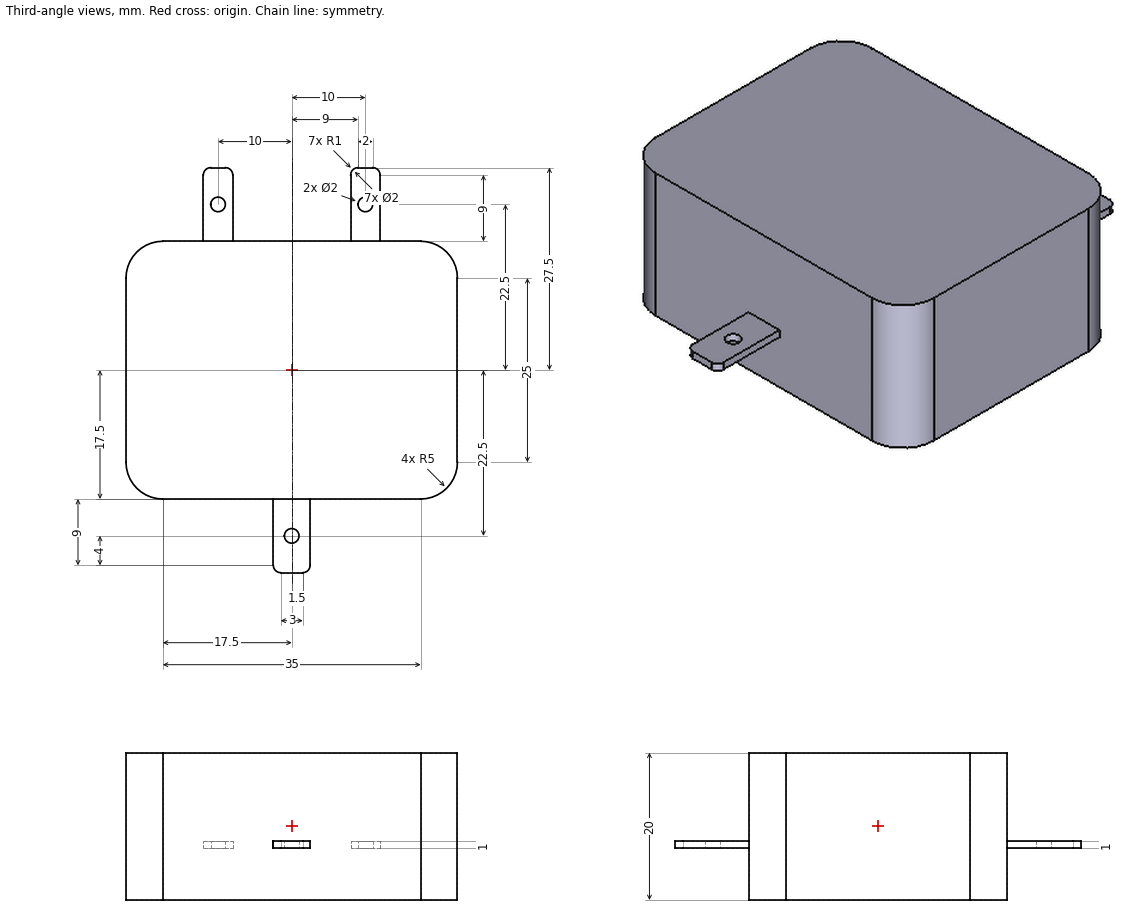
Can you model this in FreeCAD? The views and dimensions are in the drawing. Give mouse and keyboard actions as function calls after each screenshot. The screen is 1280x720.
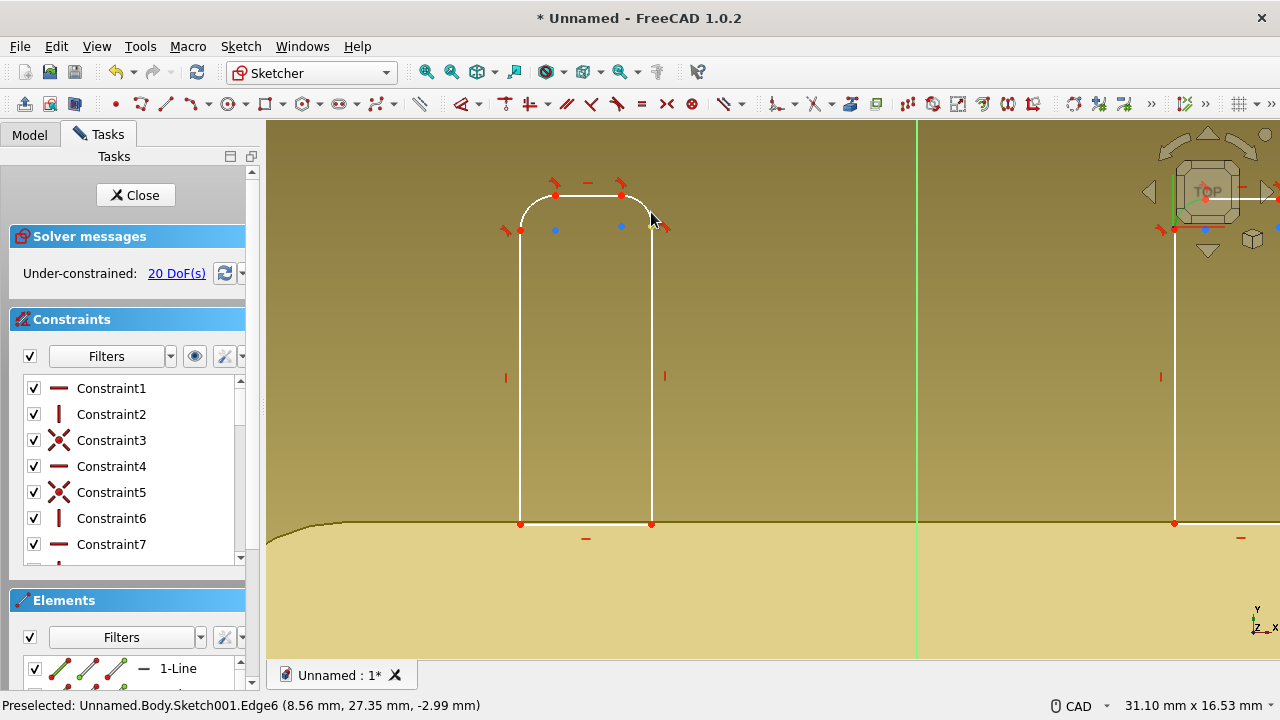
click(649, 212)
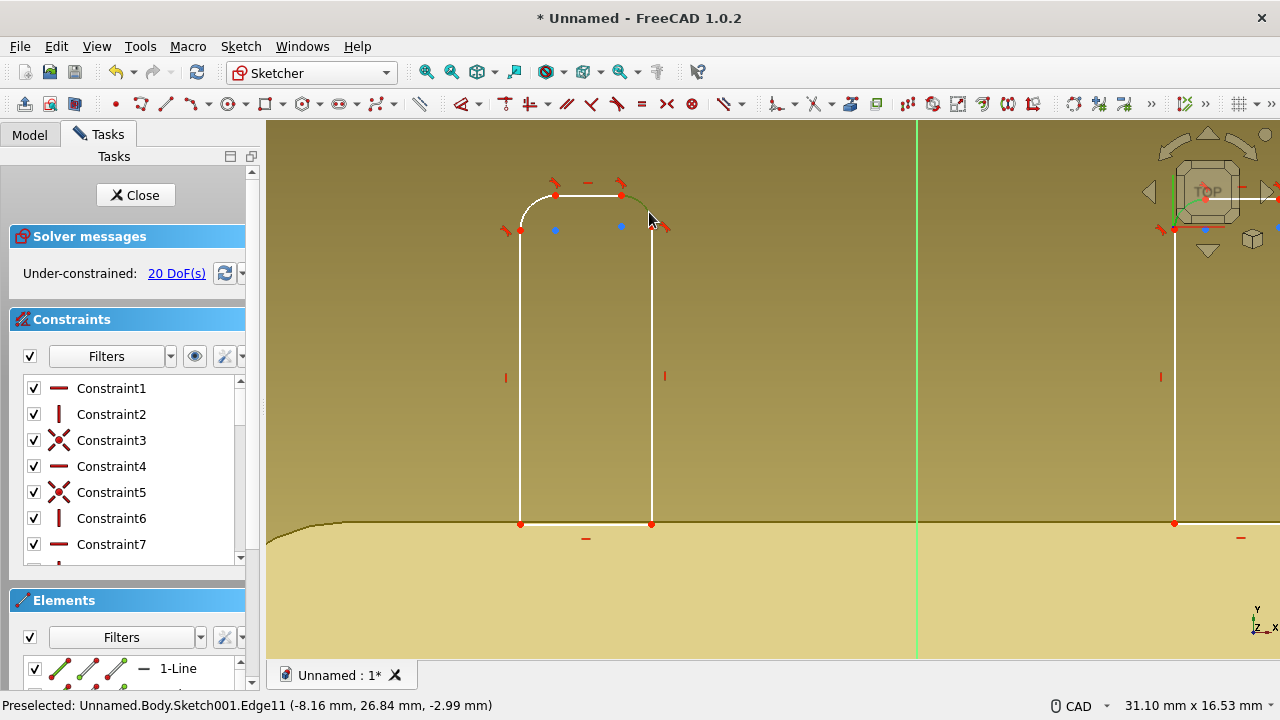
click(540, 200)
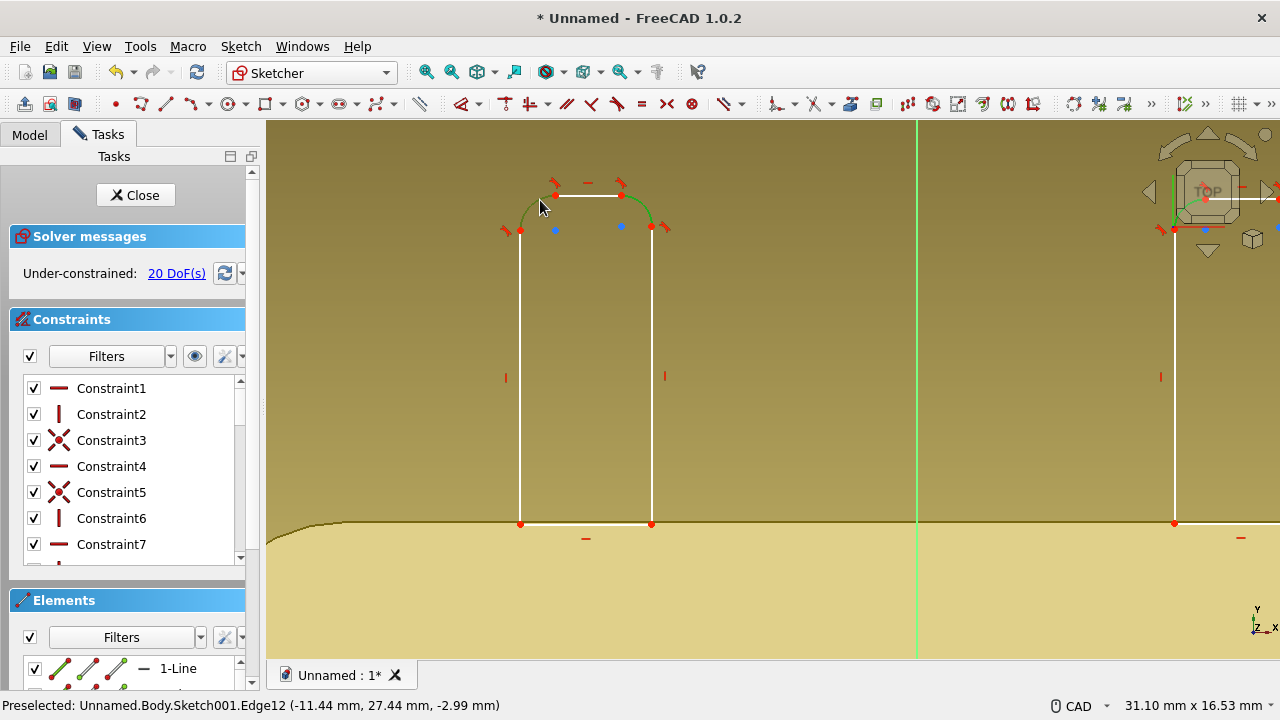
scroll(651, 212, down, 8)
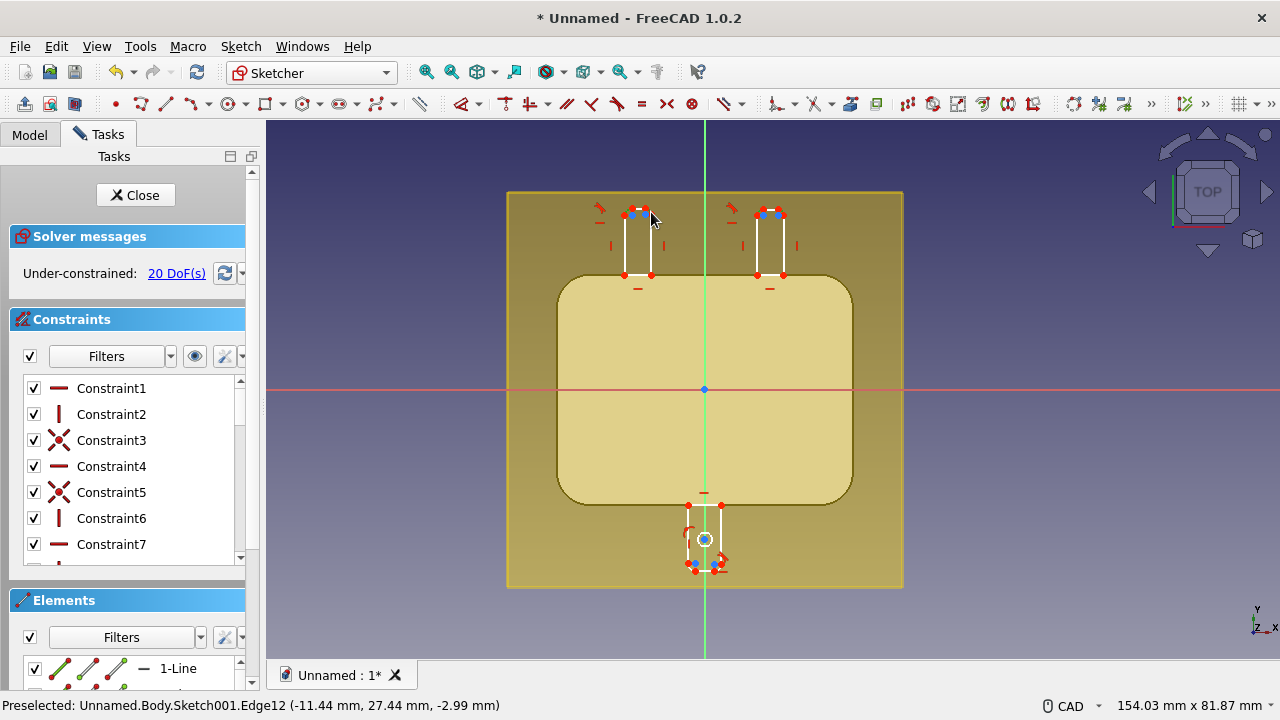
scroll(689, 567, up, 7)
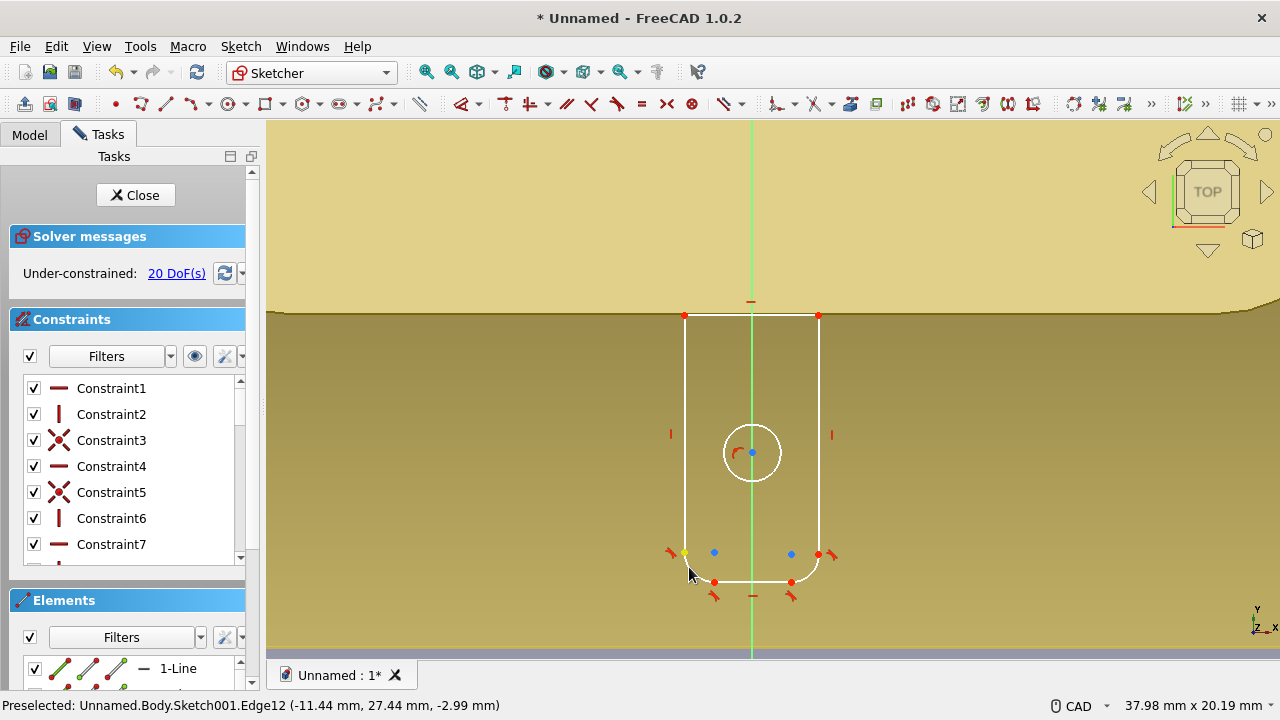
click(688, 566)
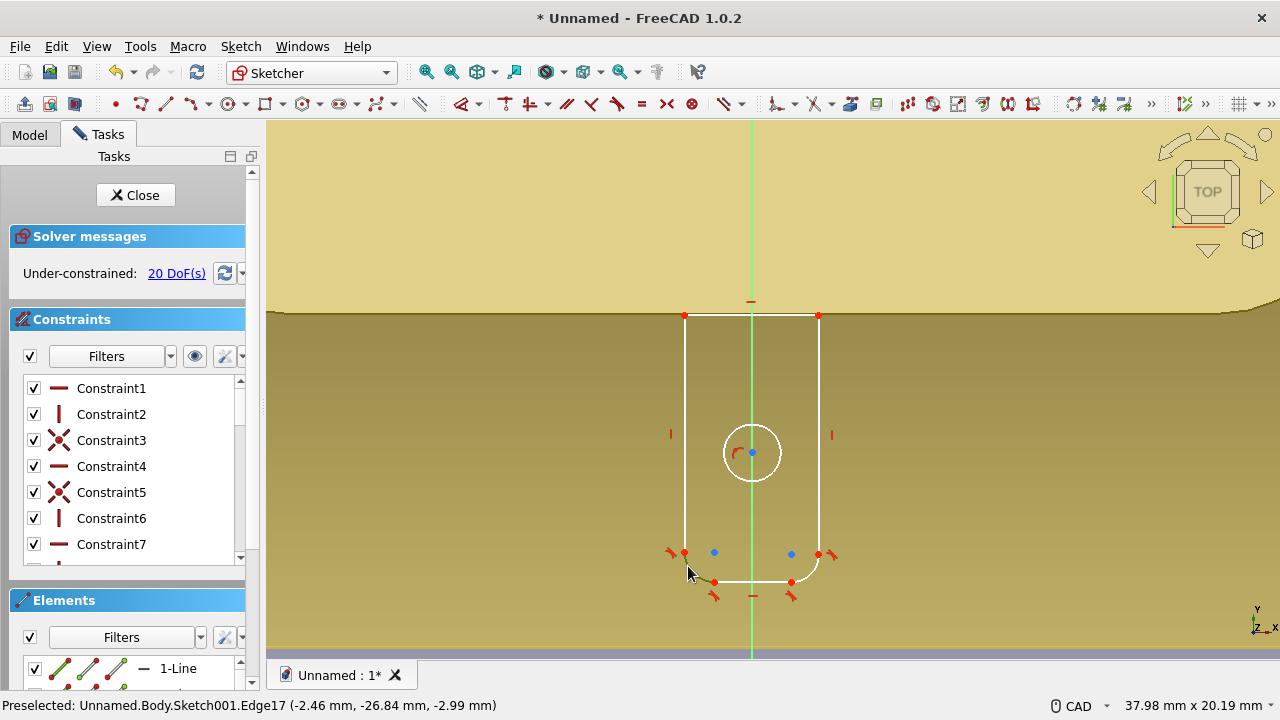
click(804, 579)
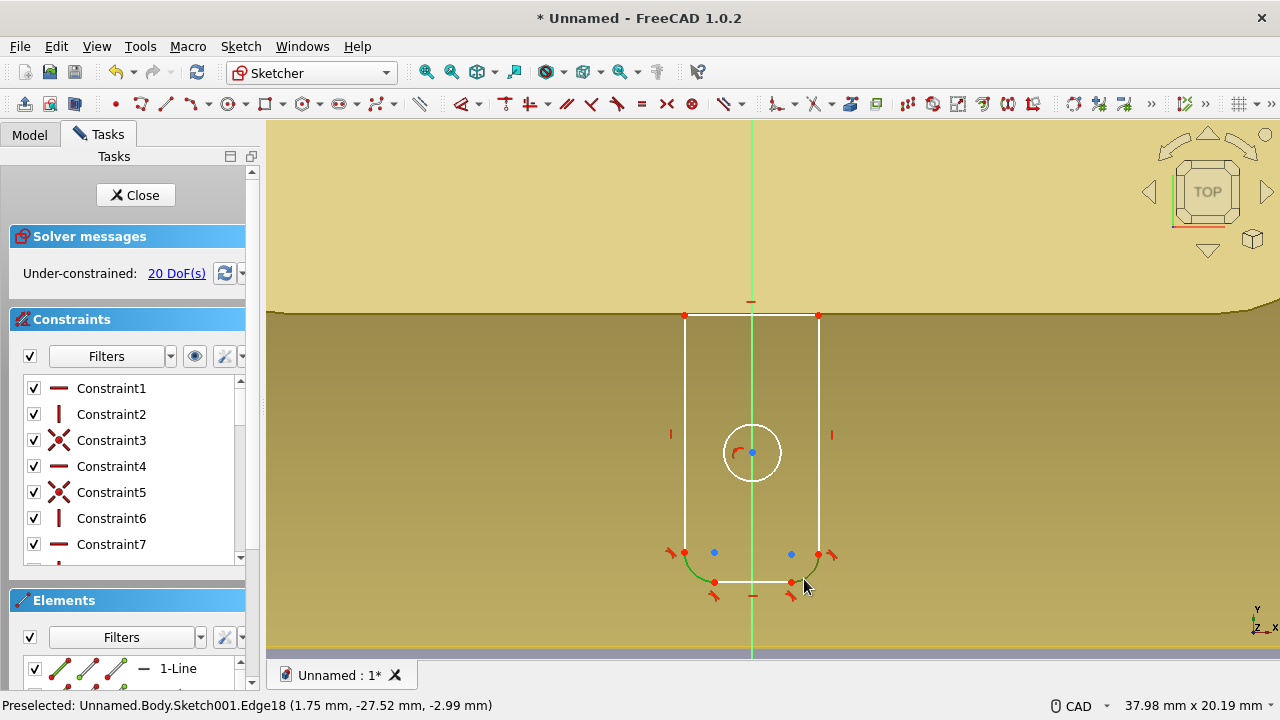
click(642, 104)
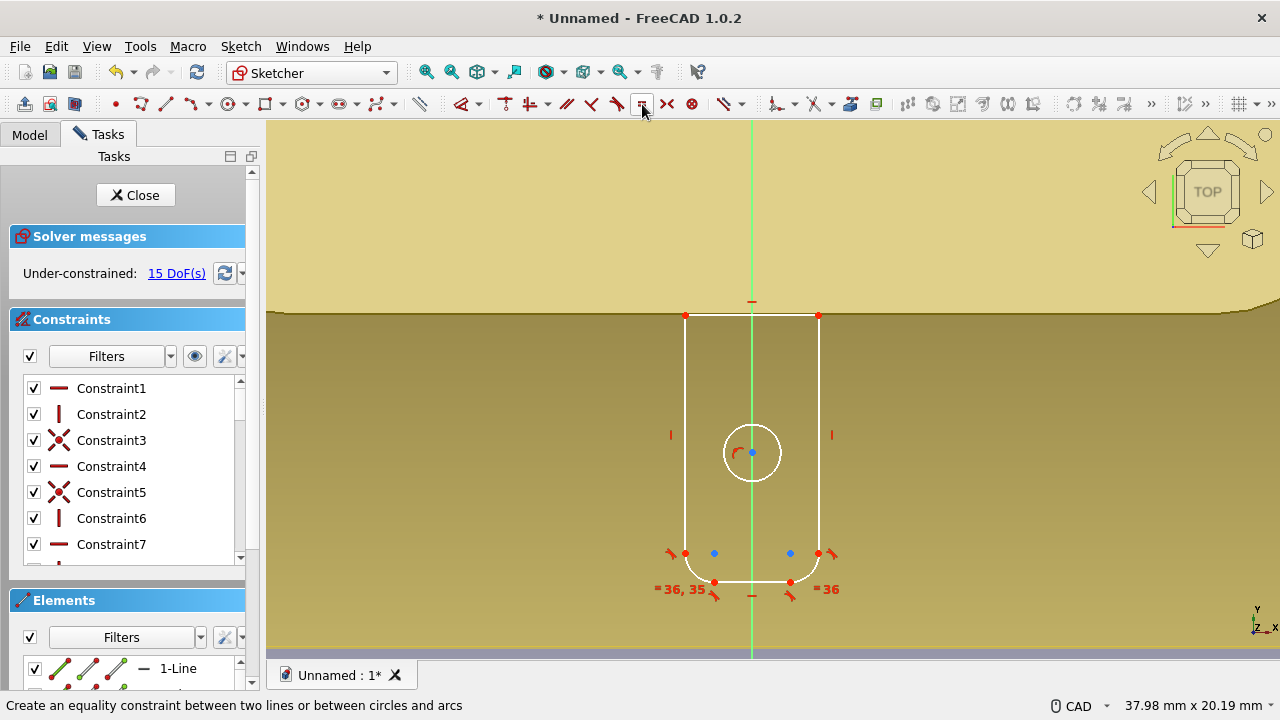
scroll(689, 567, down, 7)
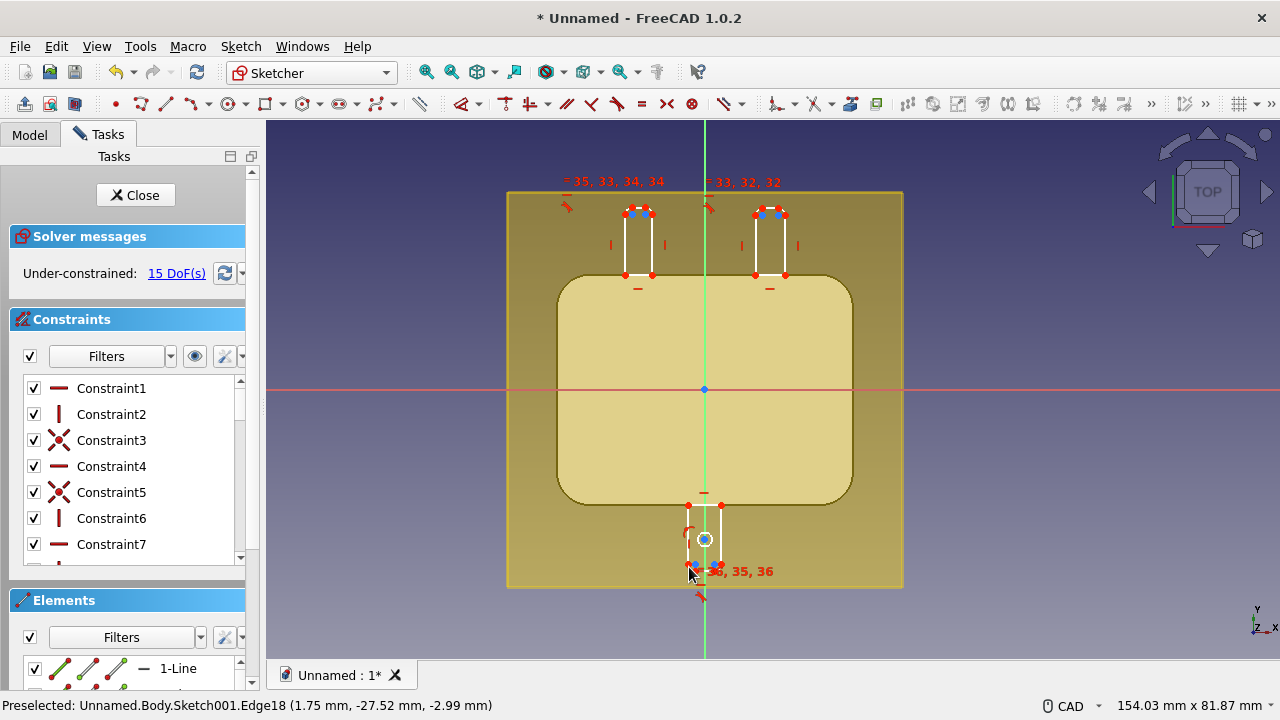
scroll(763, 215, up, 3)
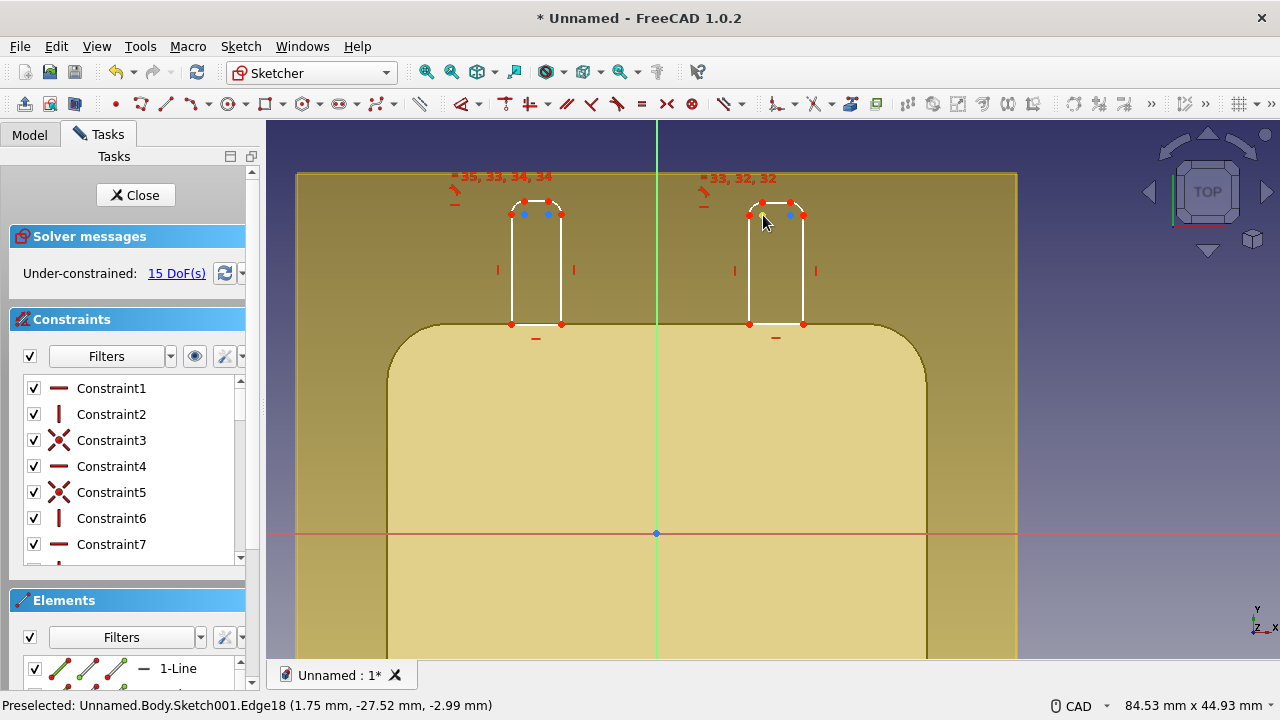
click(762, 216)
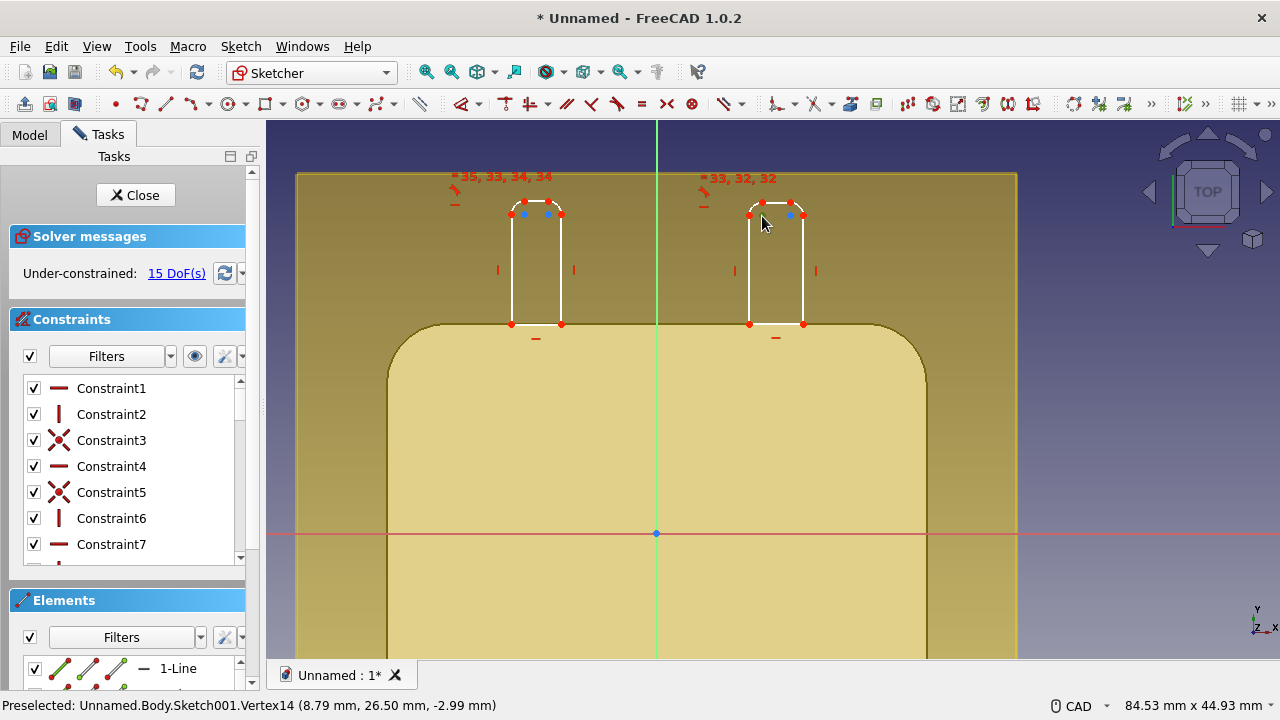
click(548, 214)